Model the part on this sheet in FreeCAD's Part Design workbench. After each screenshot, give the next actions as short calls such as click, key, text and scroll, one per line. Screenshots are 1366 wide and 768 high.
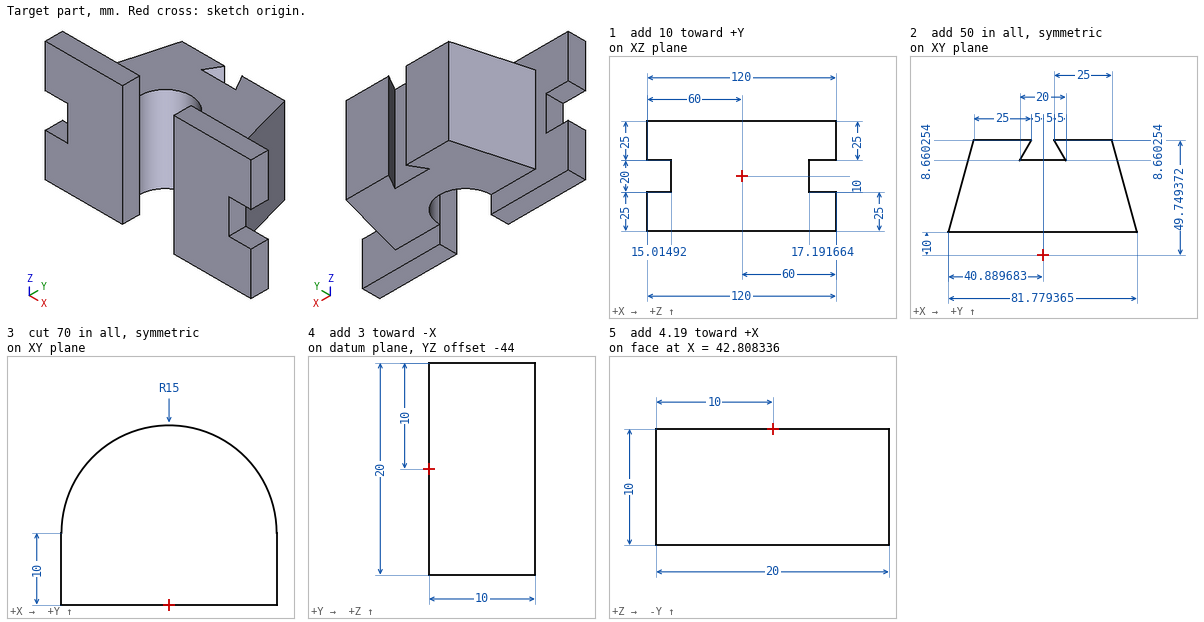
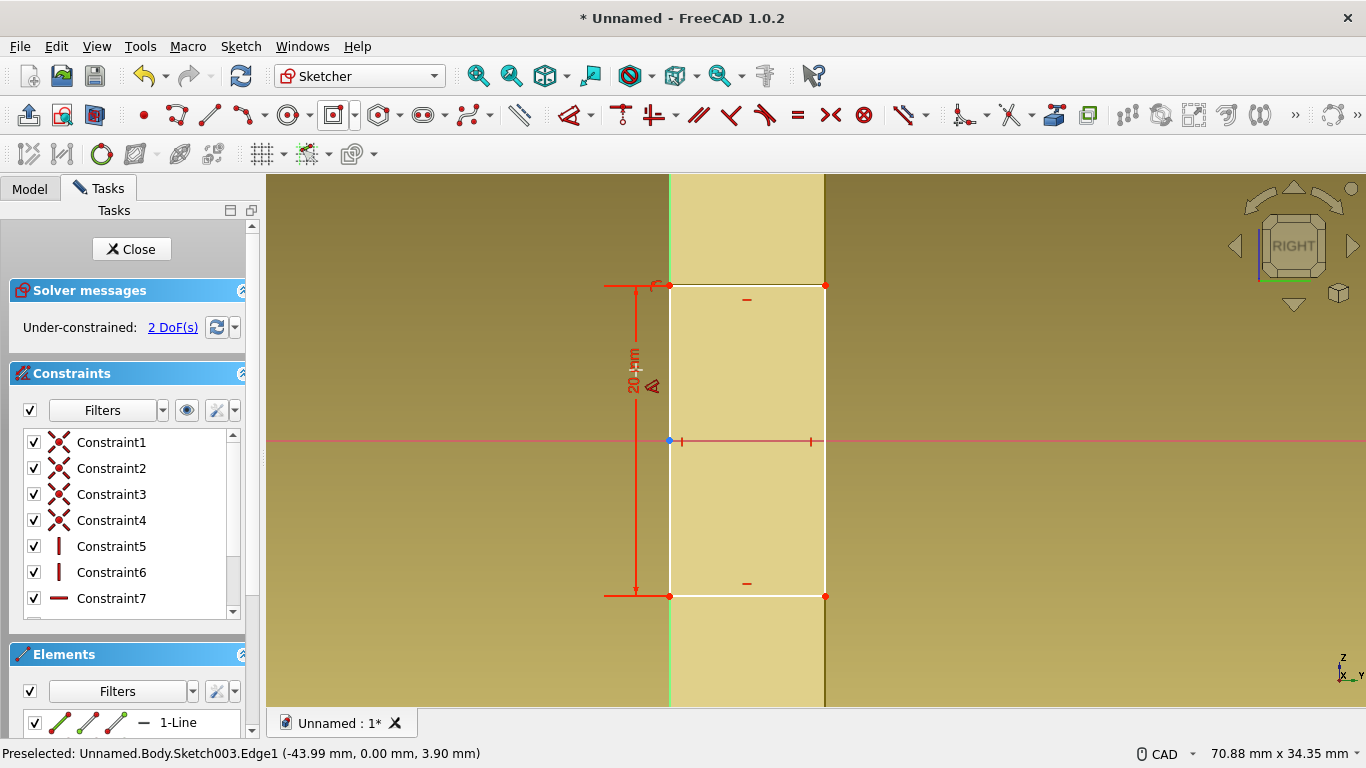
click(716, 596)
click(747, 630)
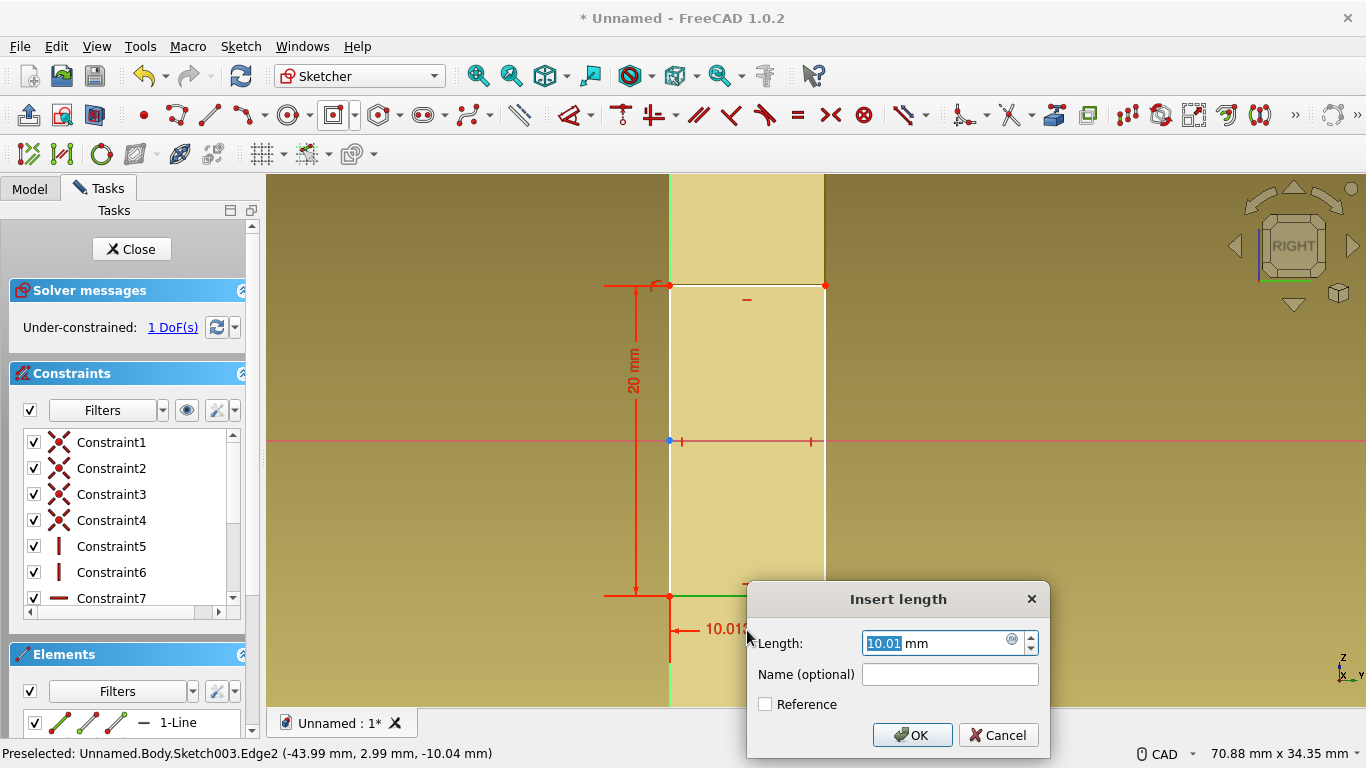
text(10)
key(Return)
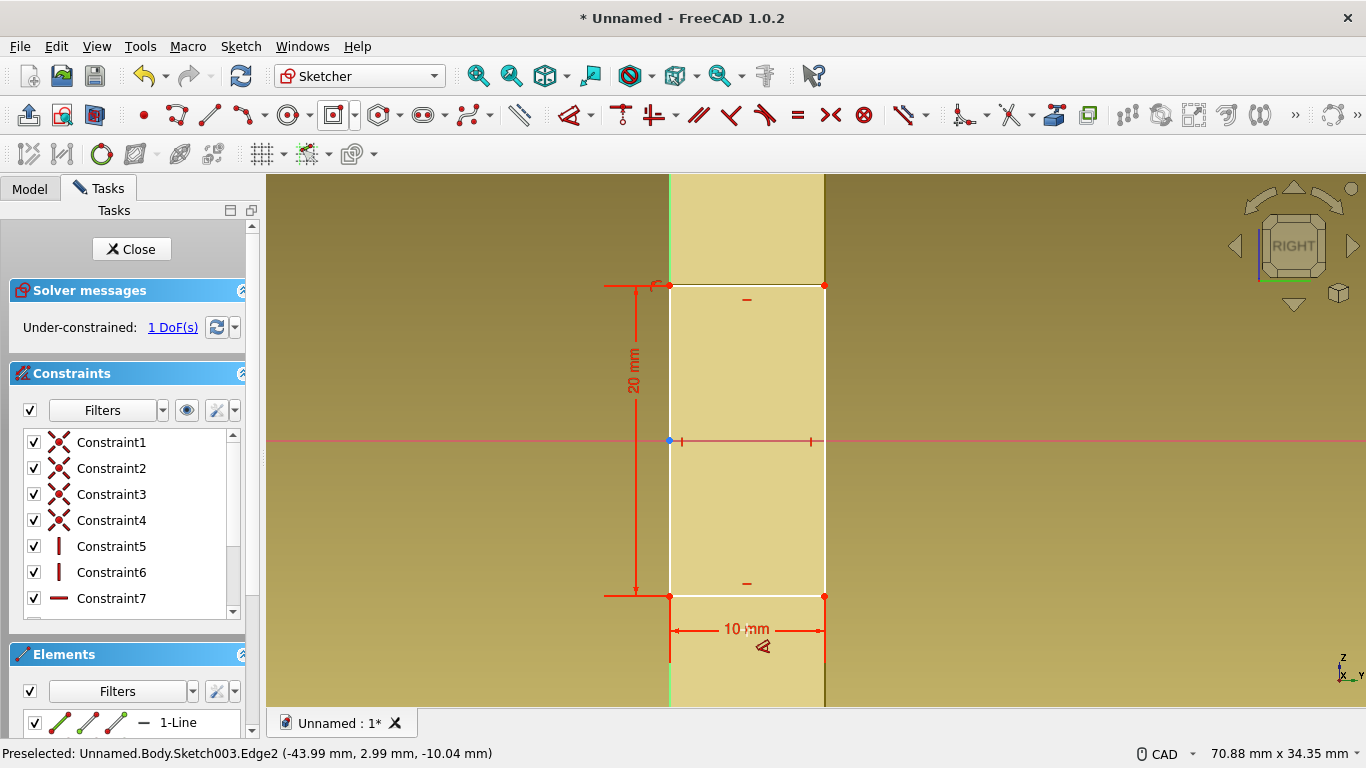
click(670, 286)
click(636, 328)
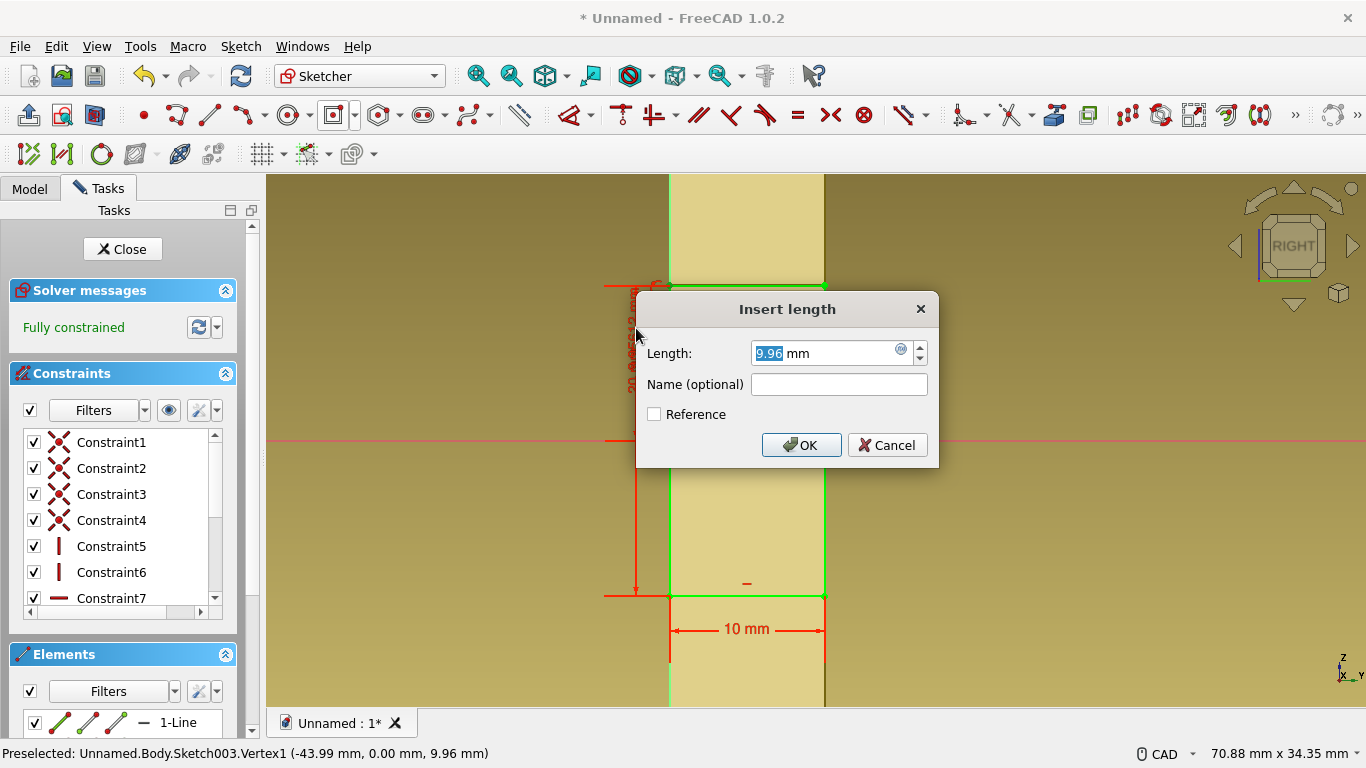
text(10)
key(Return)
key(Escape)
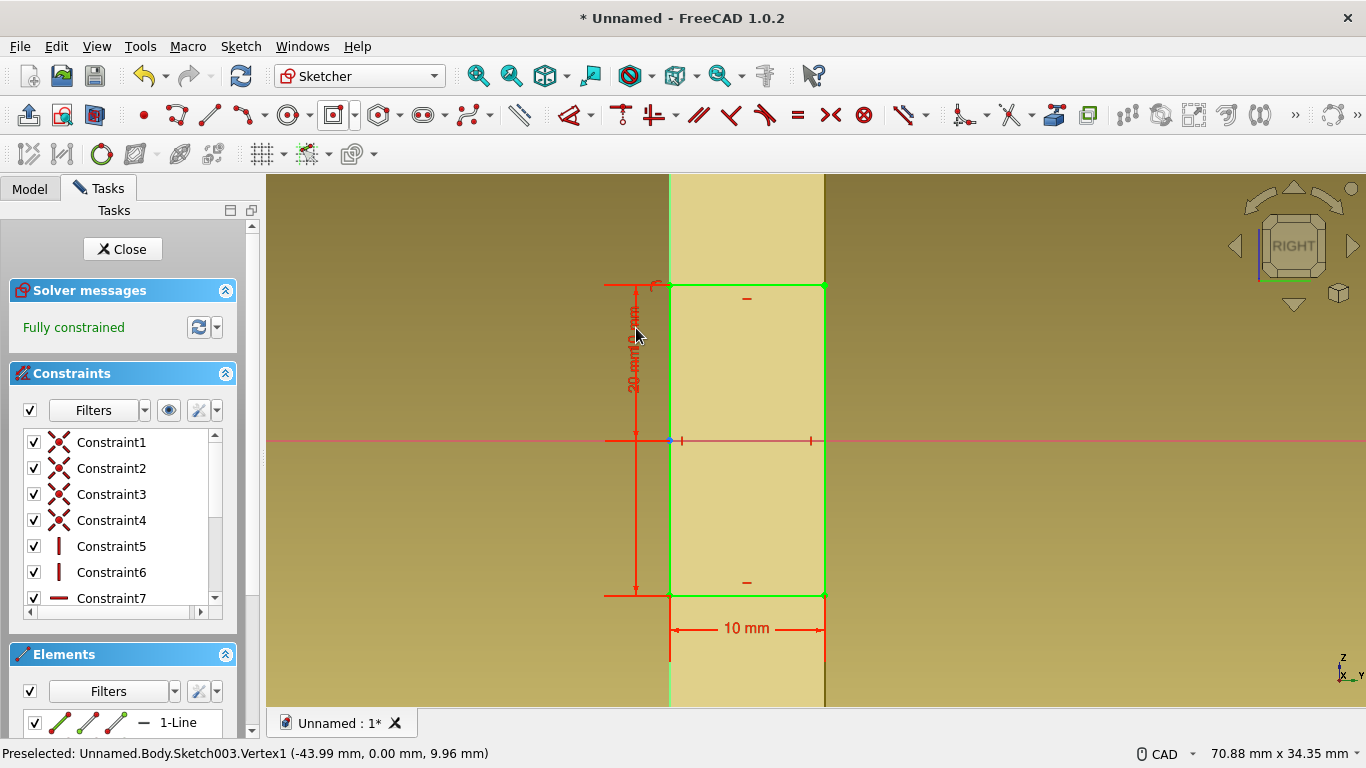
click(123, 249)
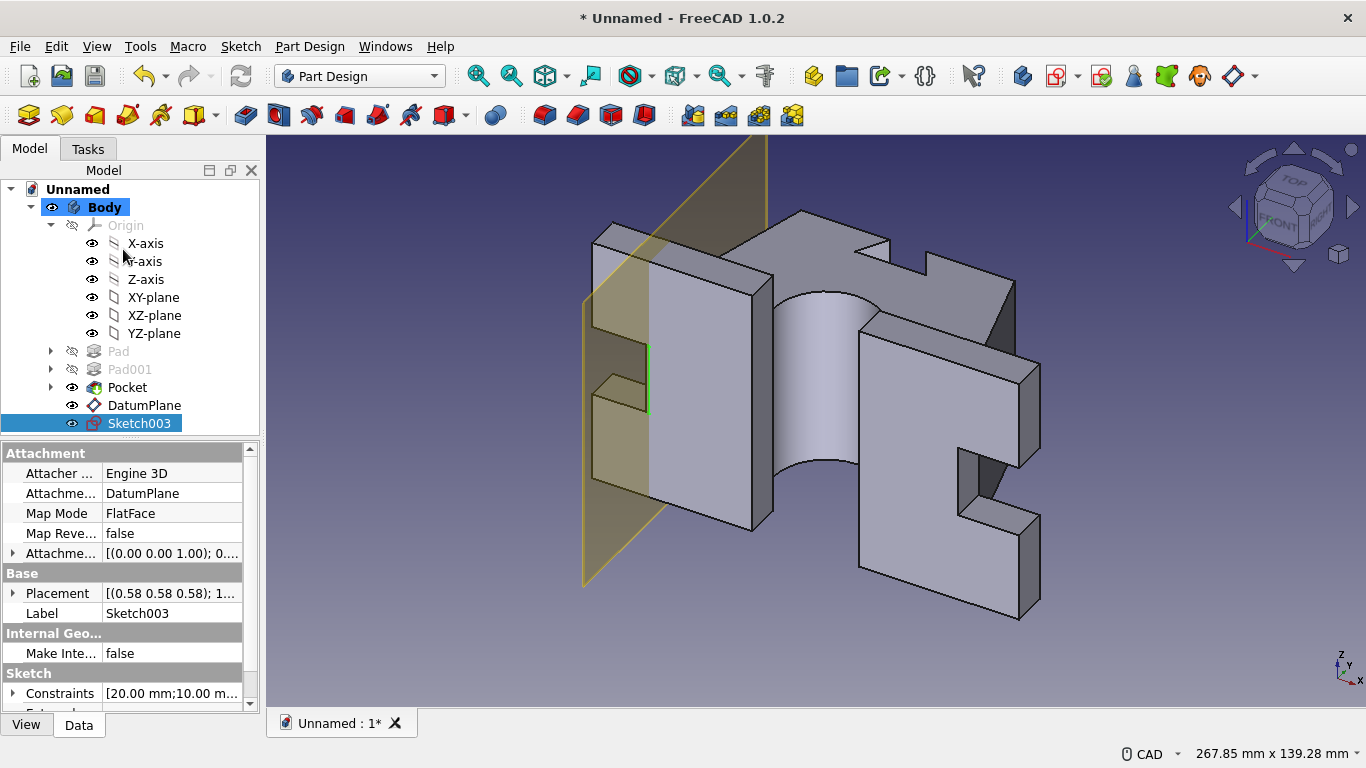
click(29, 116)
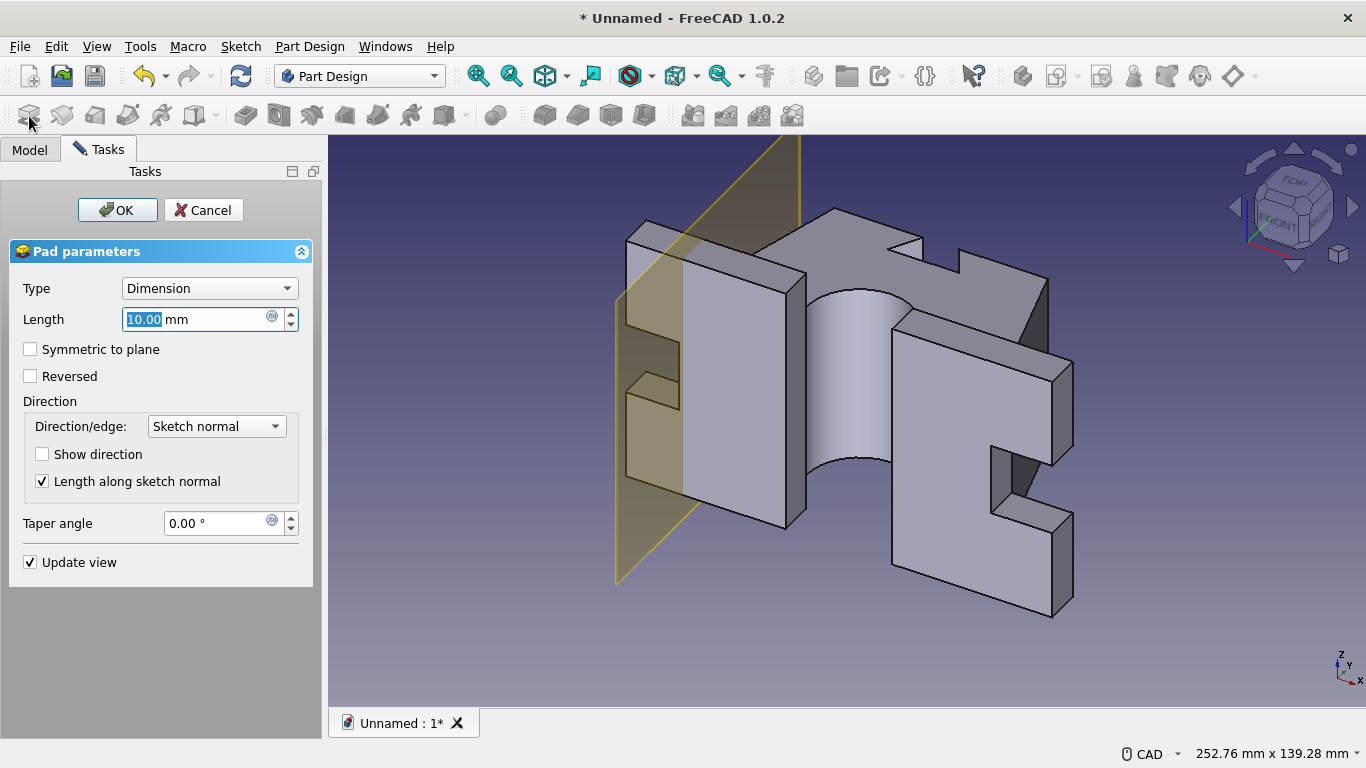
text(3)
key(Tab)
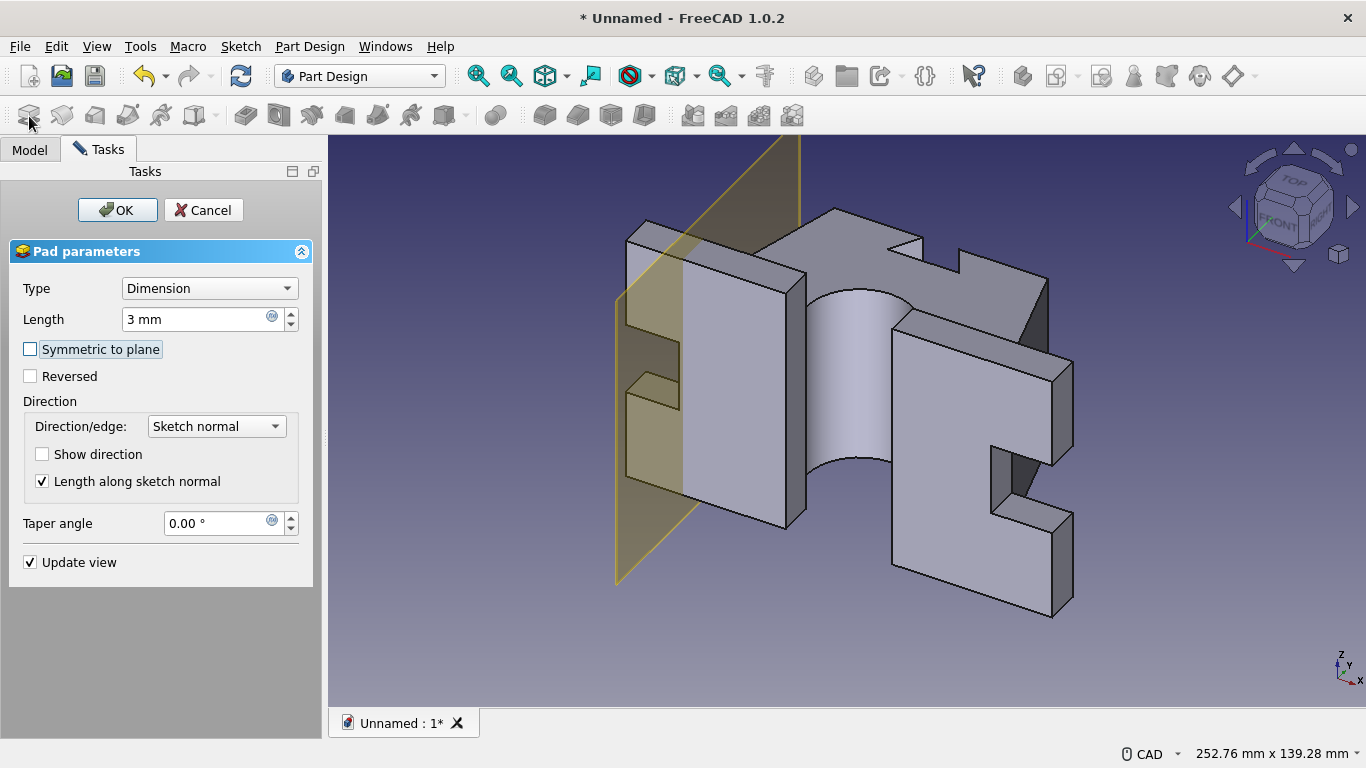
click(31, 376)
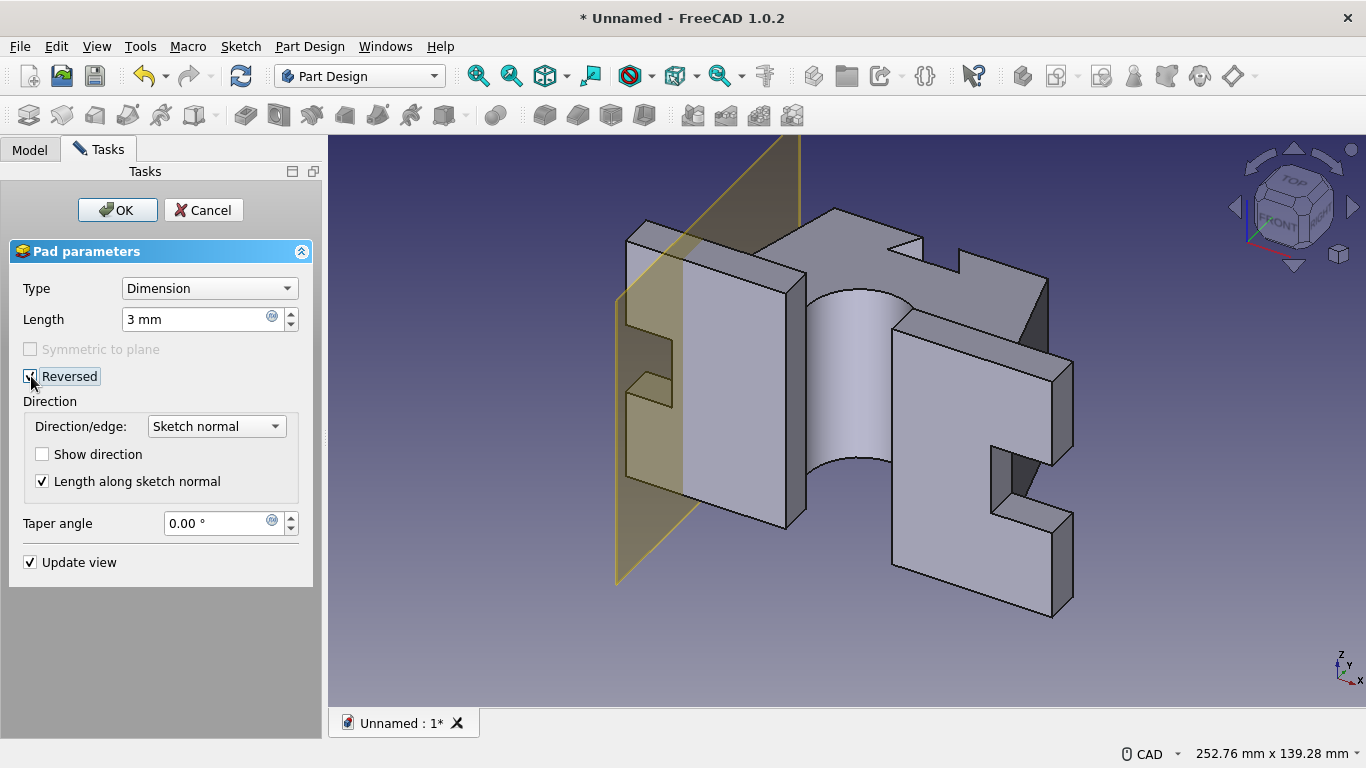
click(118, 210)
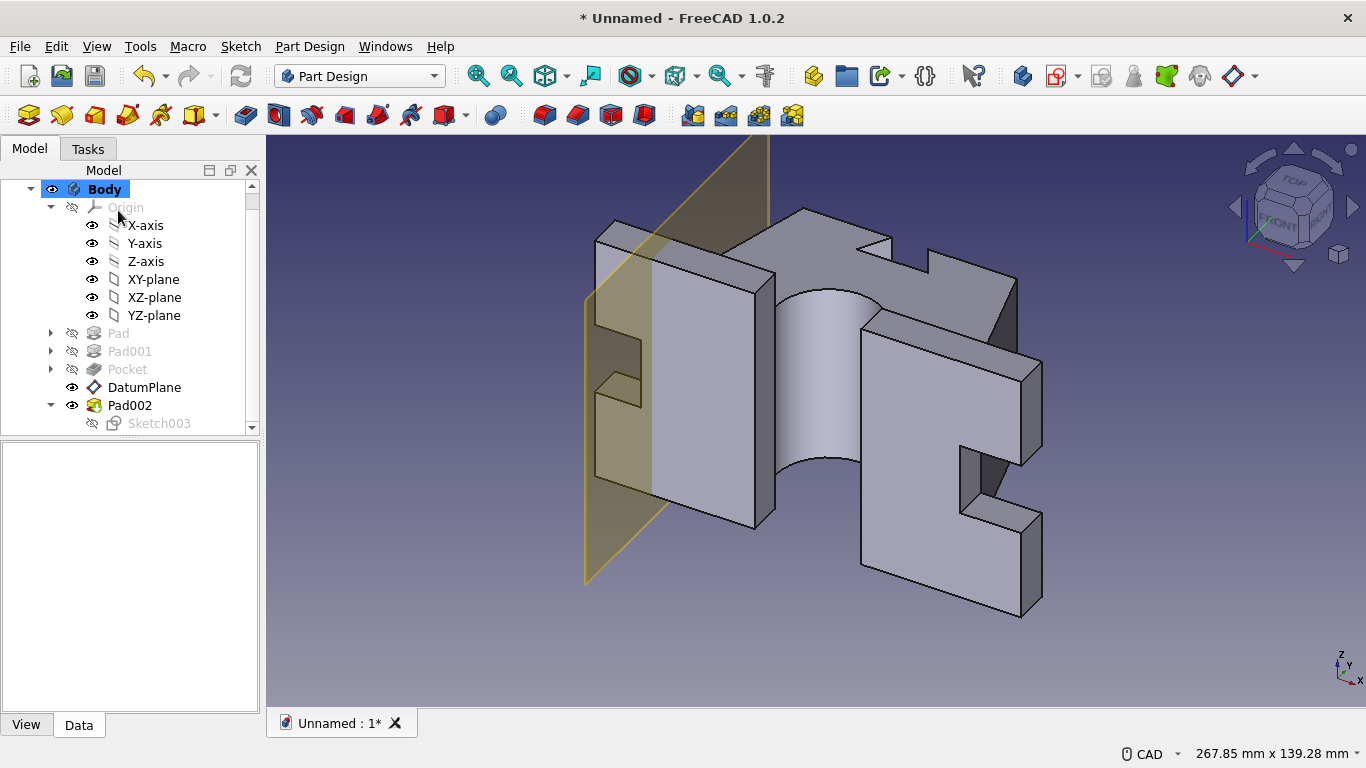
click(117, 387)
key(space)